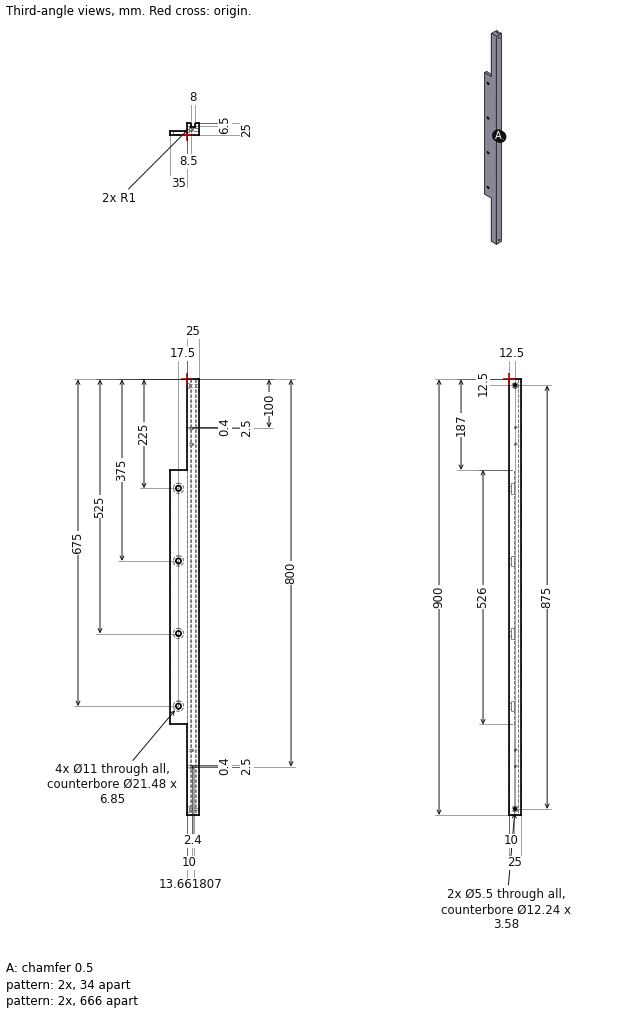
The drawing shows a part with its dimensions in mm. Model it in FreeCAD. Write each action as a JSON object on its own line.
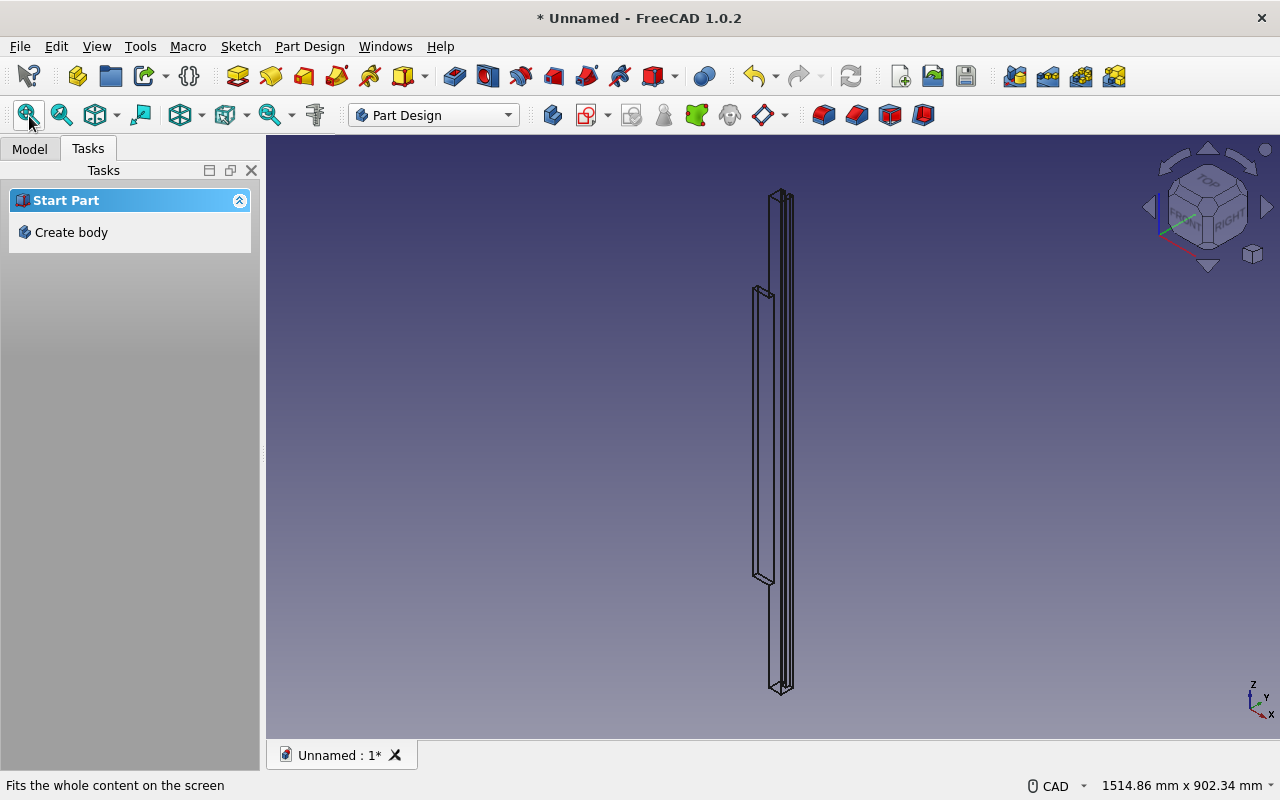
{"action": "scroll", "coordinate": [790, 439], "scroll_direction": "up", "scroll_amount": 6}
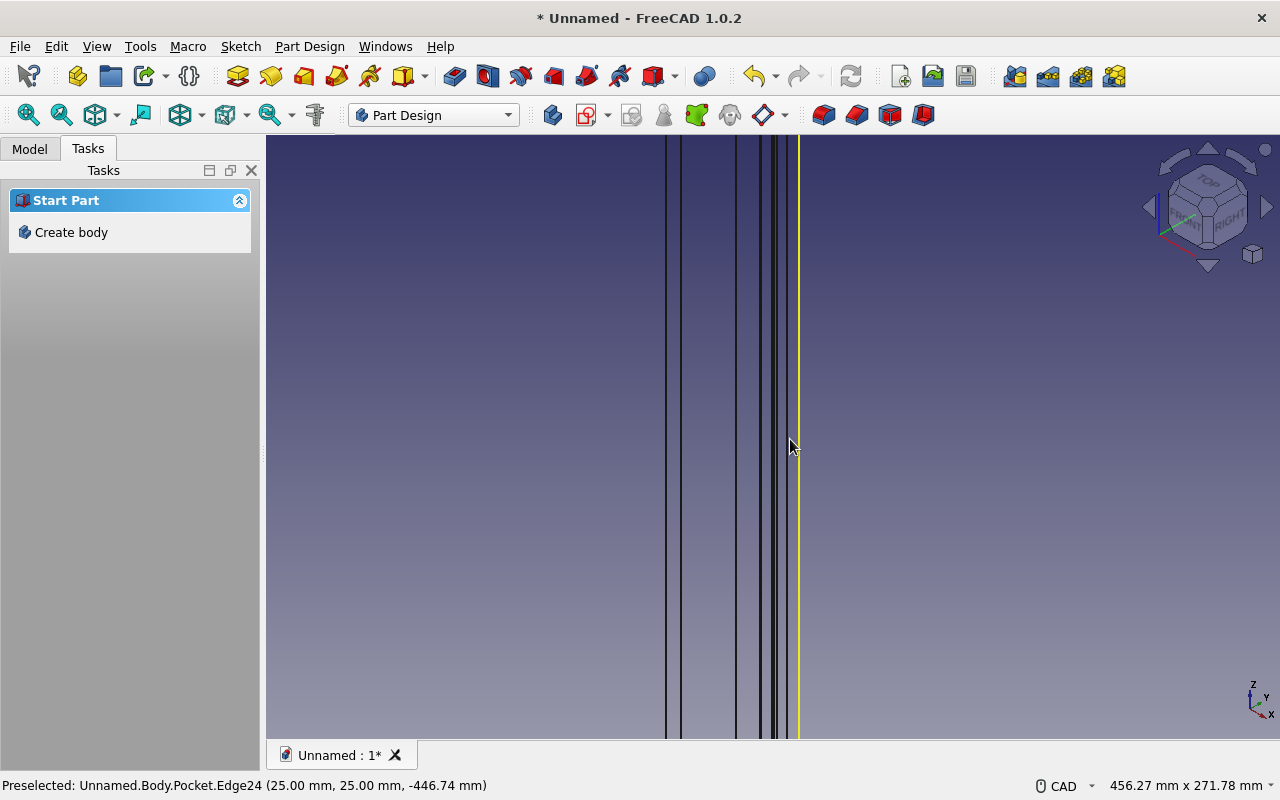
{"action": "left_click", "coordinate": [787, 439]}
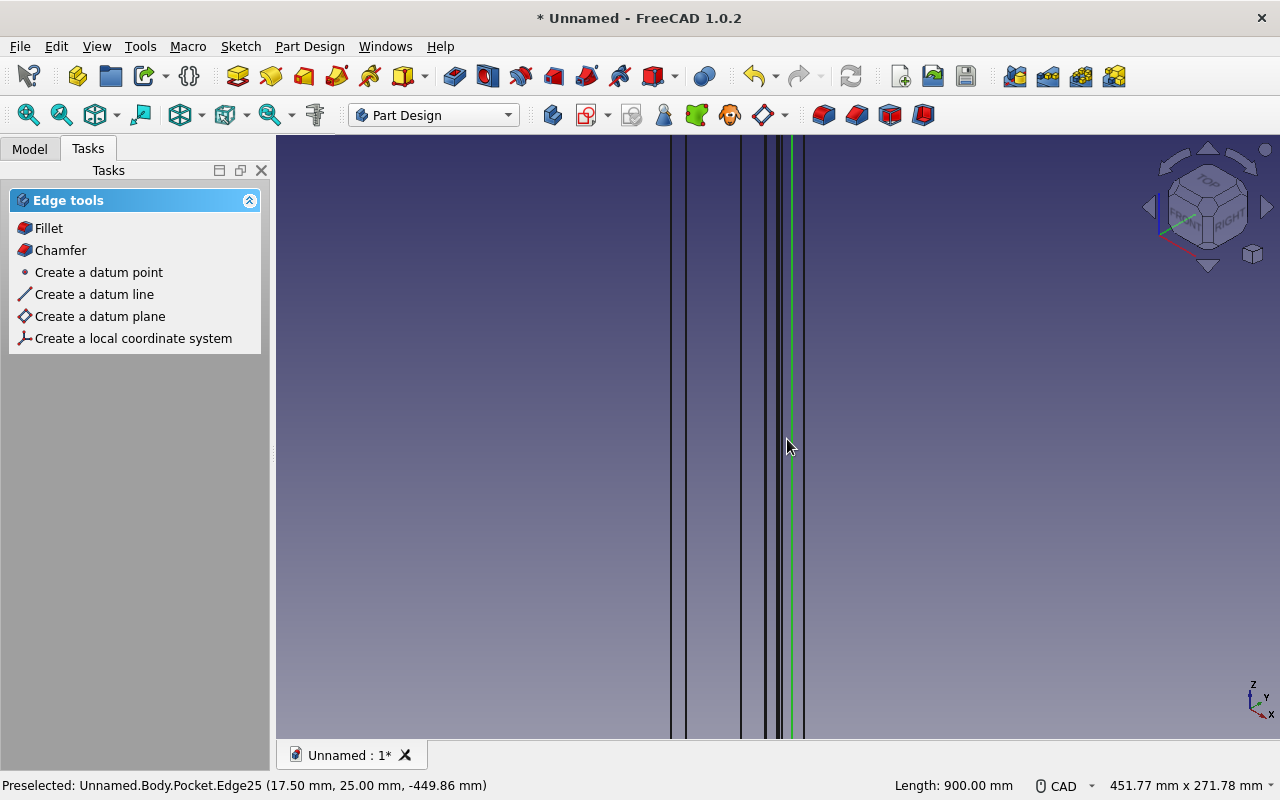
{"action": "left_click", "coordinate": [29, 116]}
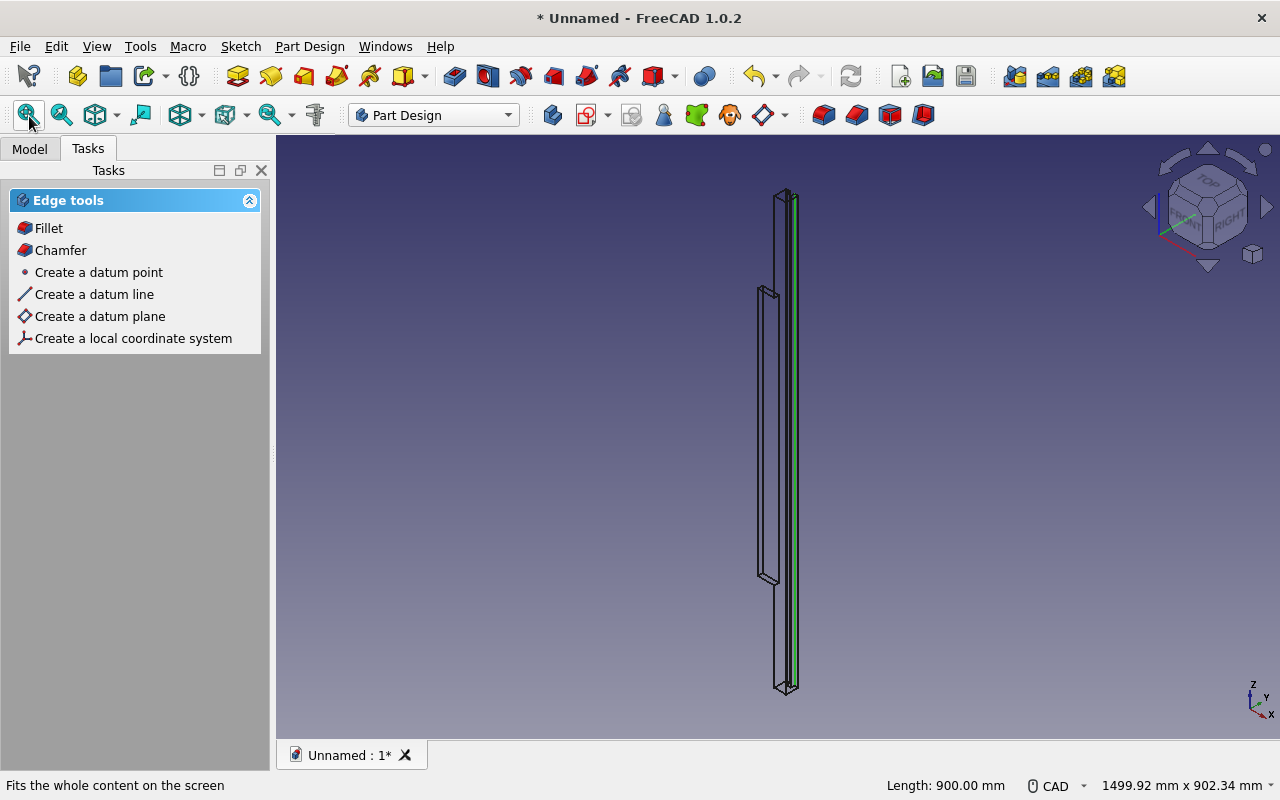
{"action": "key", "text": "2"}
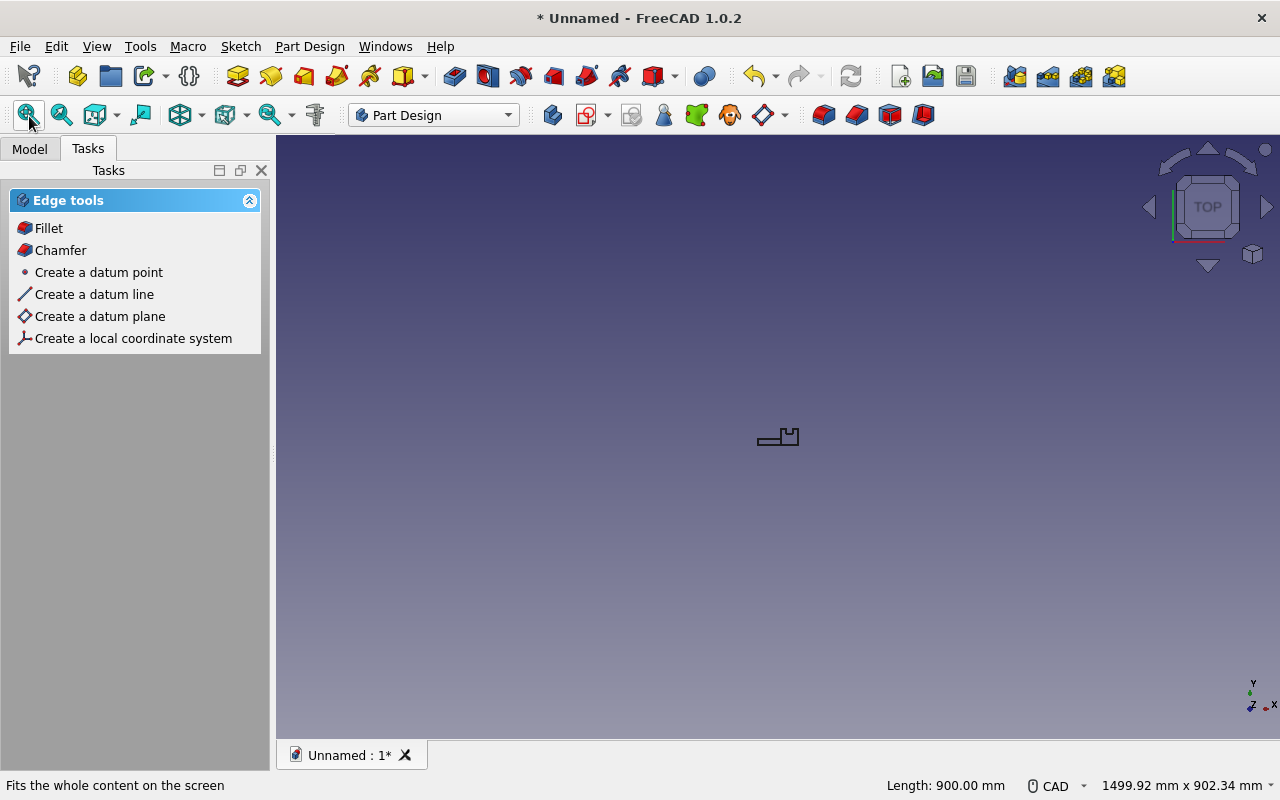
{"action": "left_click", "coordinate": [29, 116]}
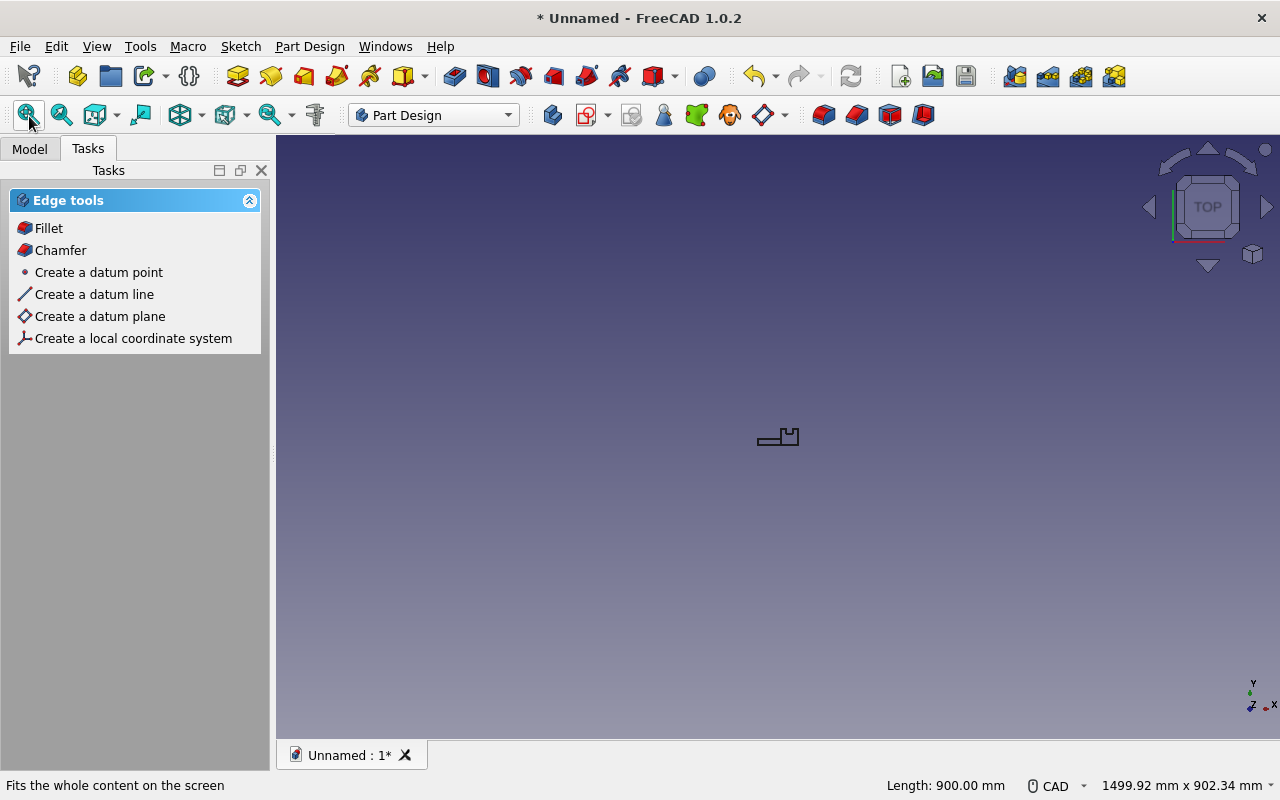
{"action": "scroll", "coordinate": [786, 428], "scroll_direction": "up", "scroll_amount": 6}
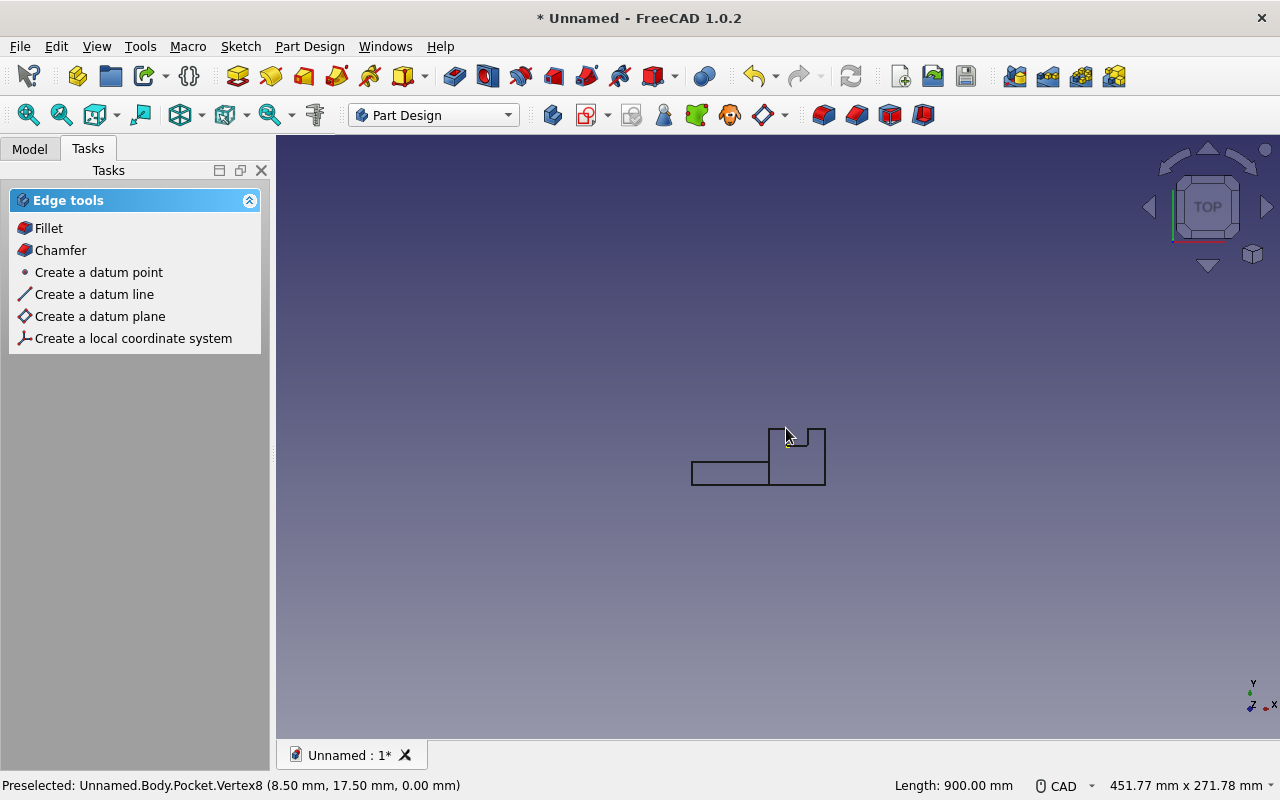
{"action": "left_click", "coordinate": [29, 116]}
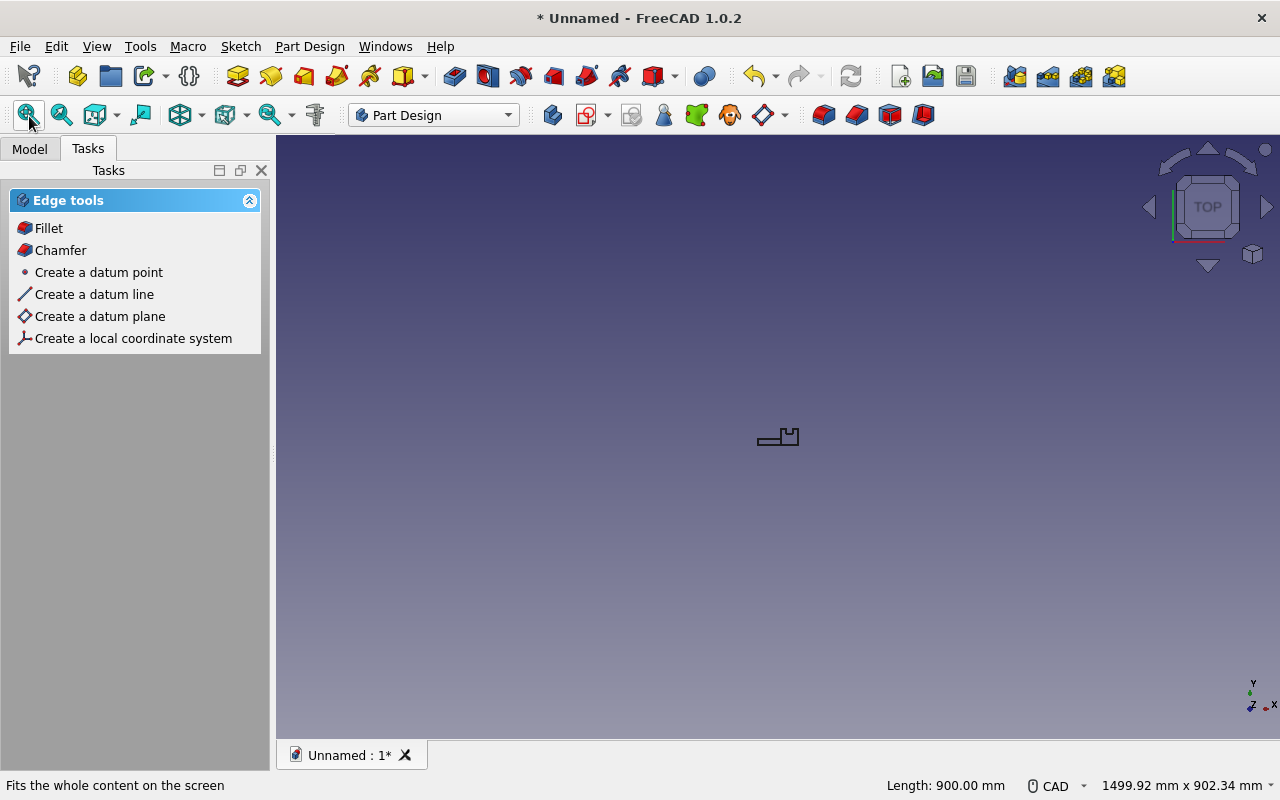
{"action": "key", "text": "1"}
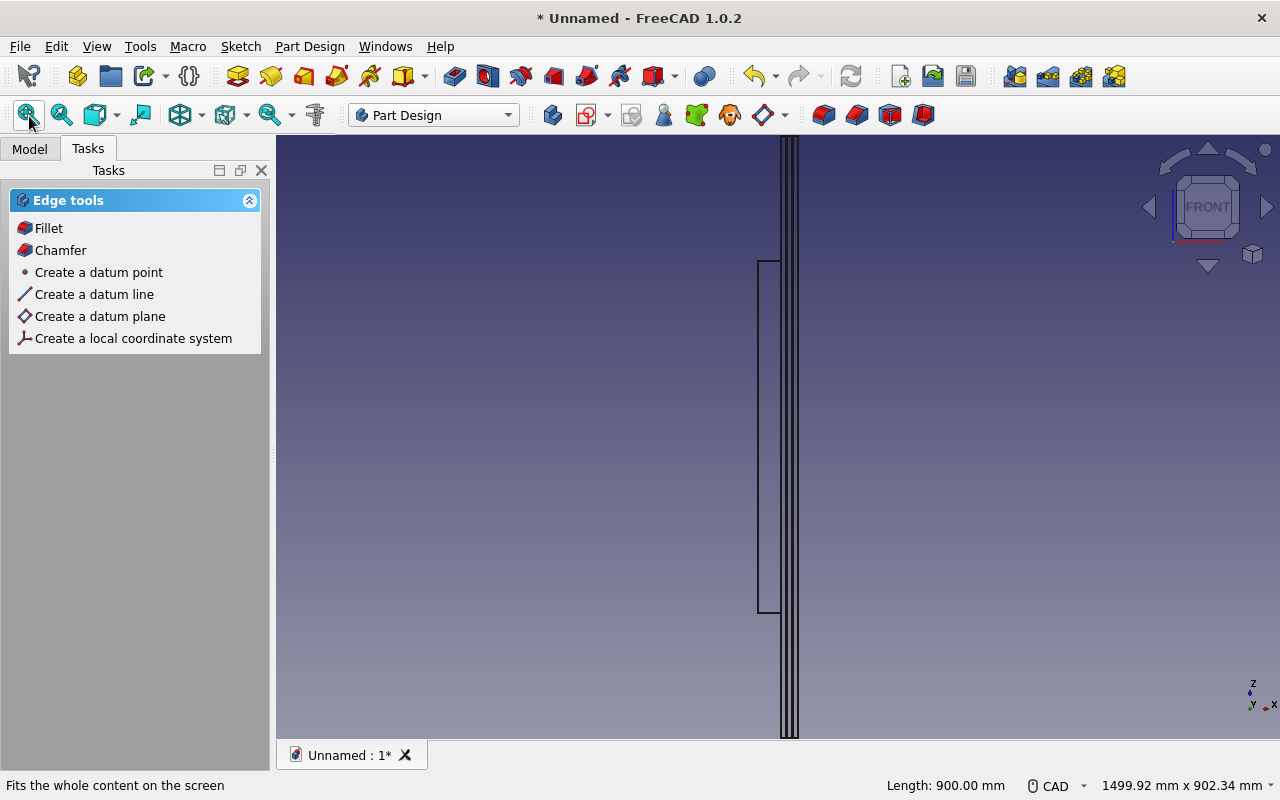
{"action": "scroll", "coordinate": [786, 436], "scroll_direction": "up", "scroll_amount": 6}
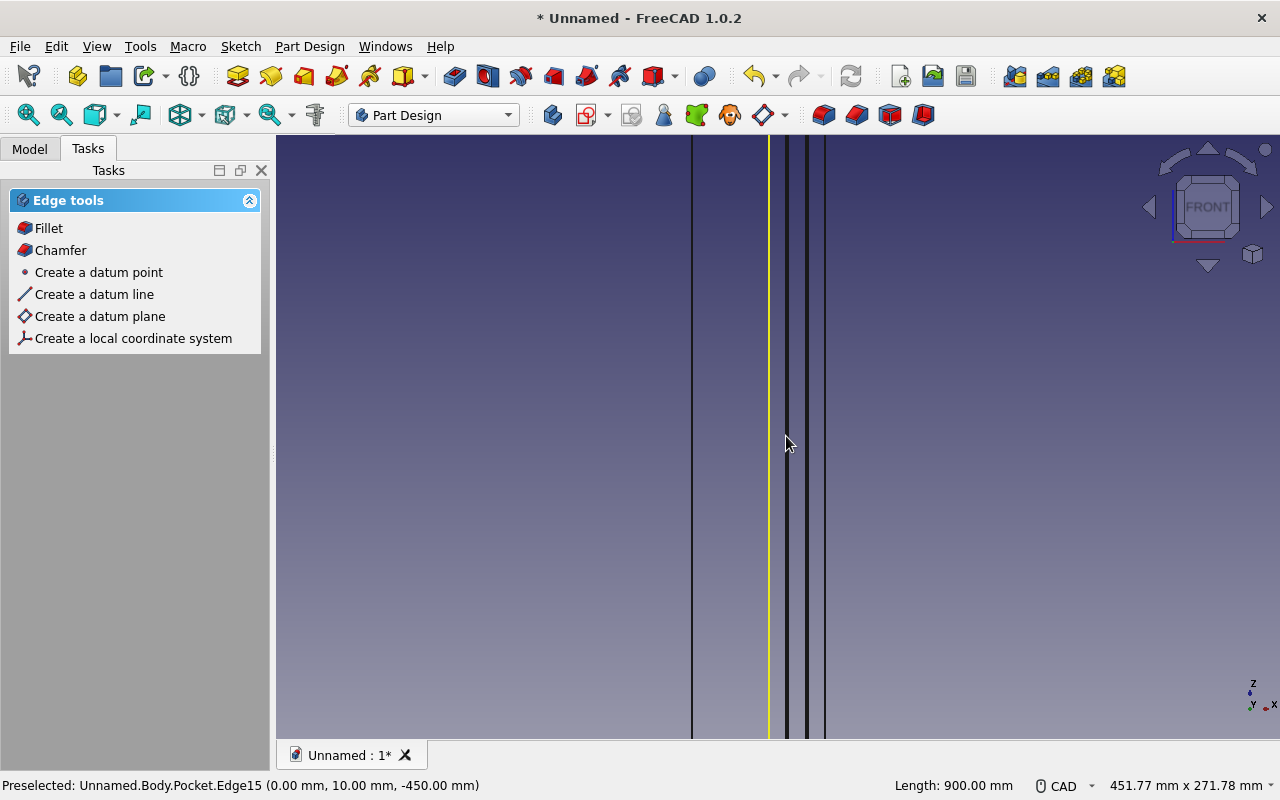
{"action": "left_click", "coordinate": [29, 116]}